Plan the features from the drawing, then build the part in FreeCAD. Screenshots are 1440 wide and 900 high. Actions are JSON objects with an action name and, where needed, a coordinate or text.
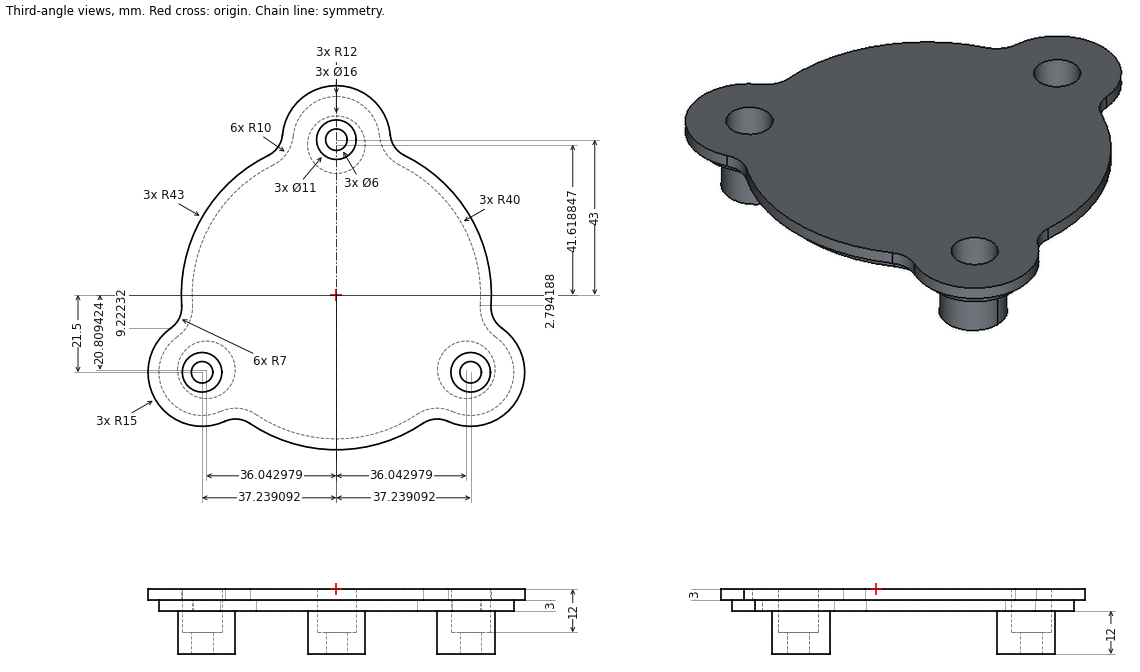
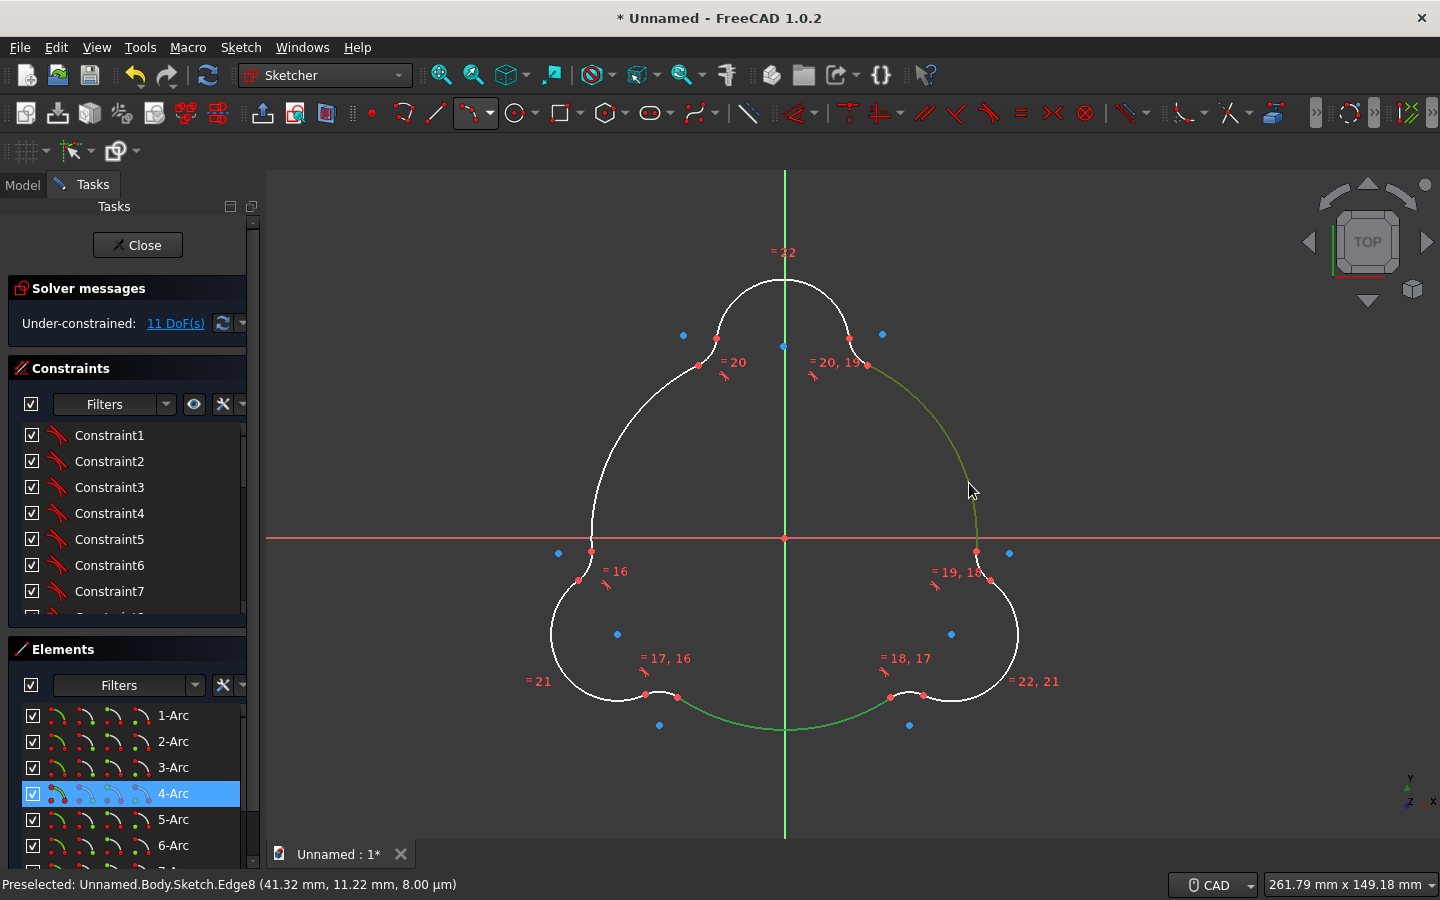
{"action": "left_click", "coordinate": [644, 406]}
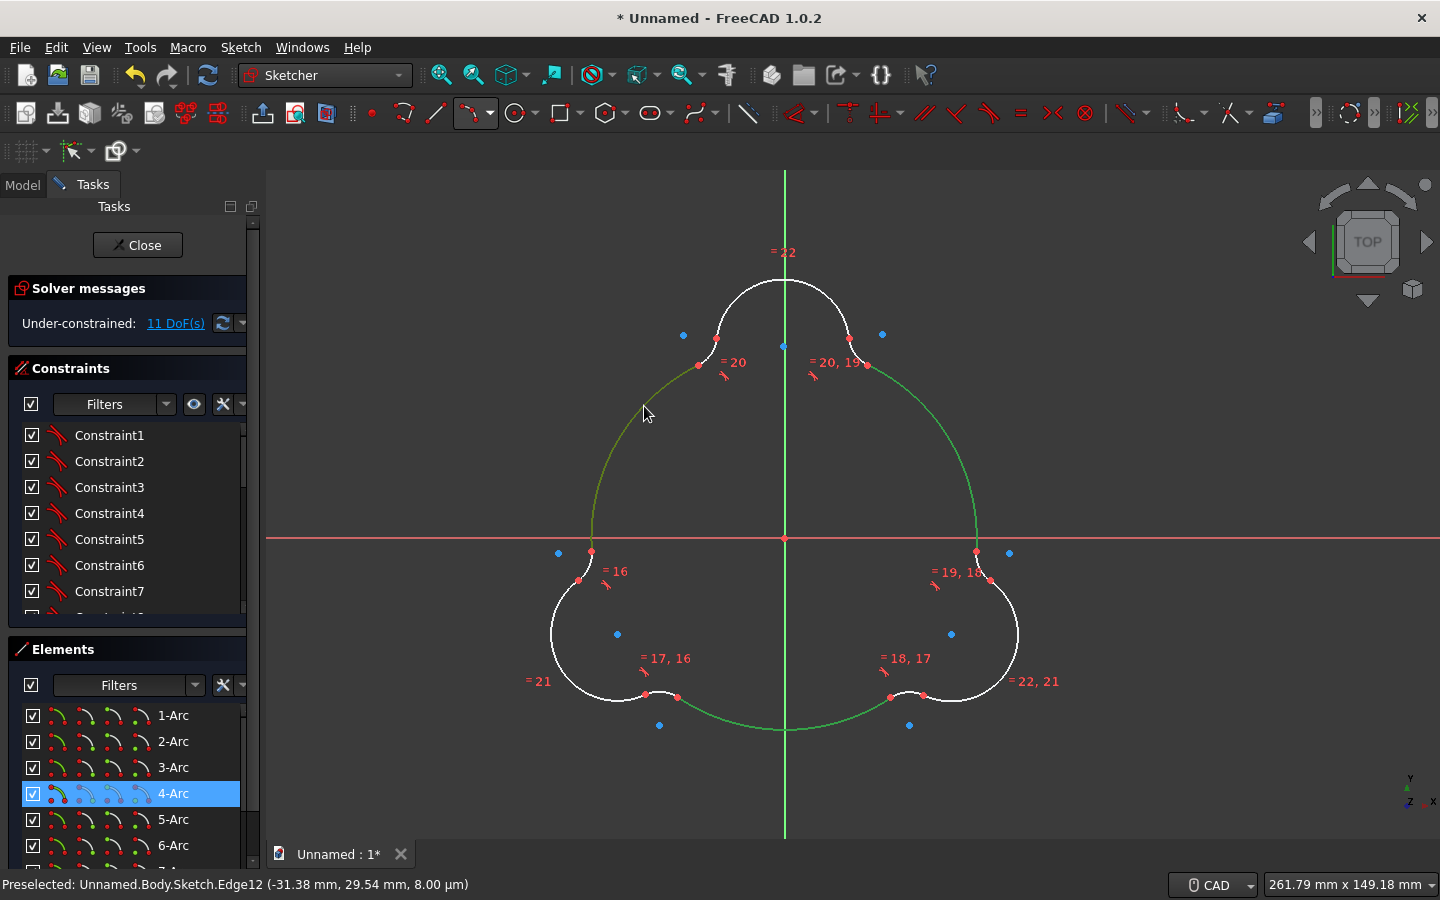
{"action": "left_click", "coordinate": [1022, 114]}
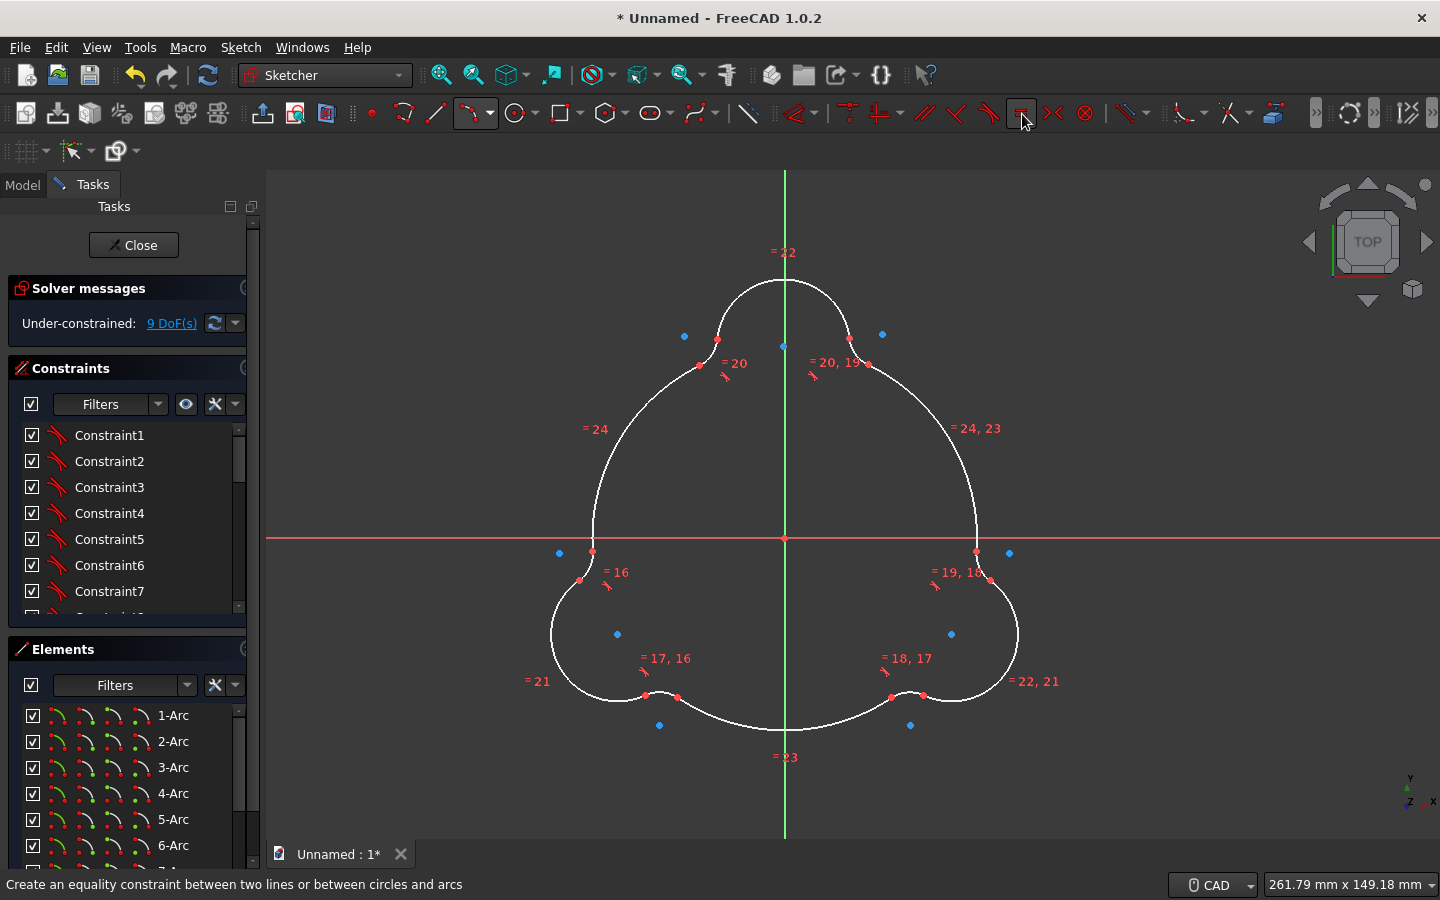
{"action": "left_click", "coordinate": [783, 346]}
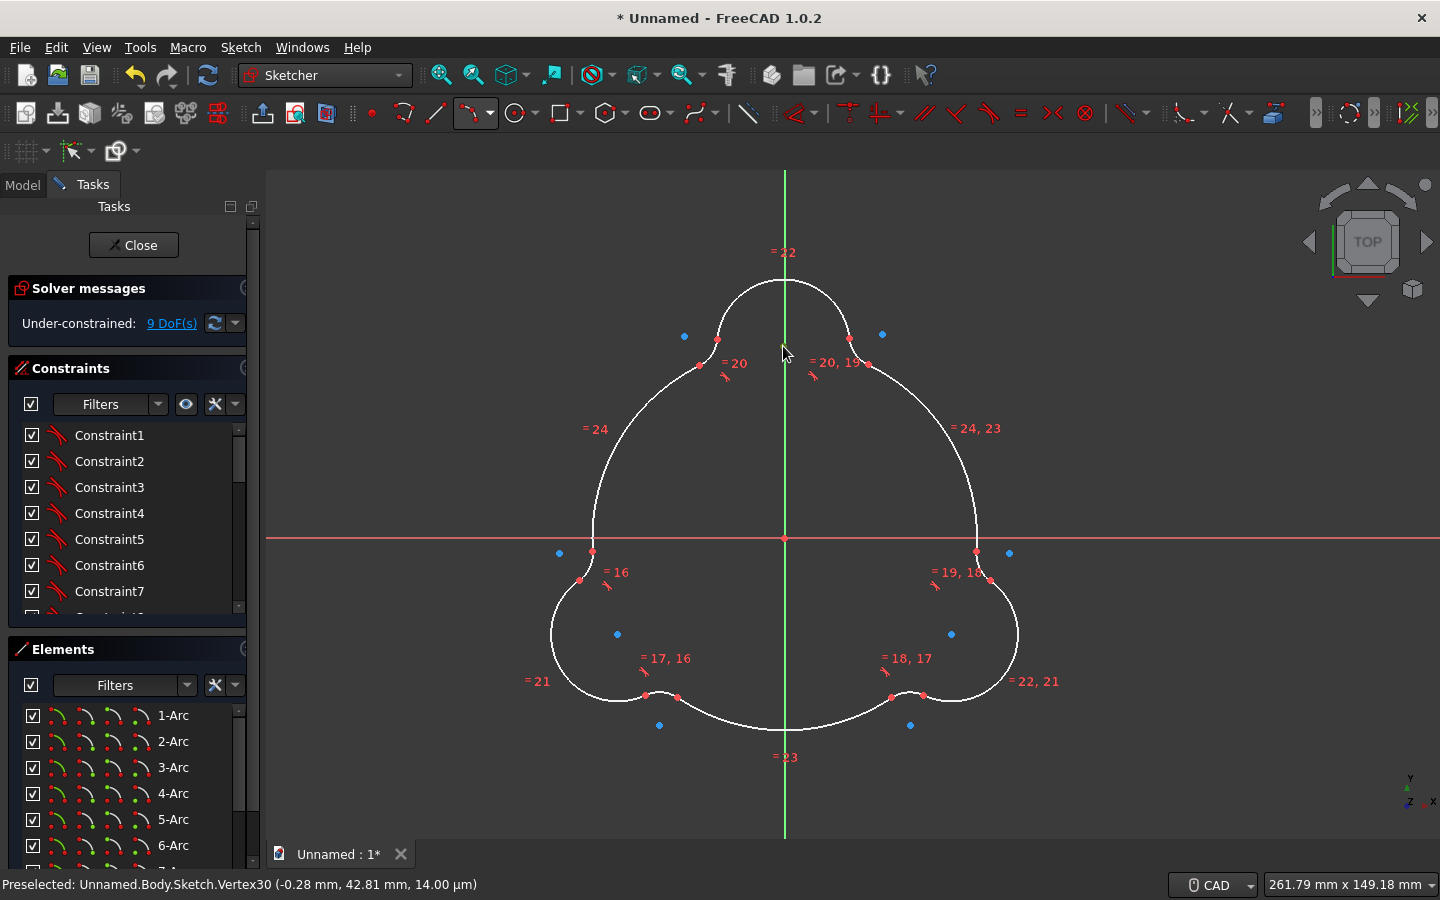
{"action": "left_click", "coordinate": [785, 767]}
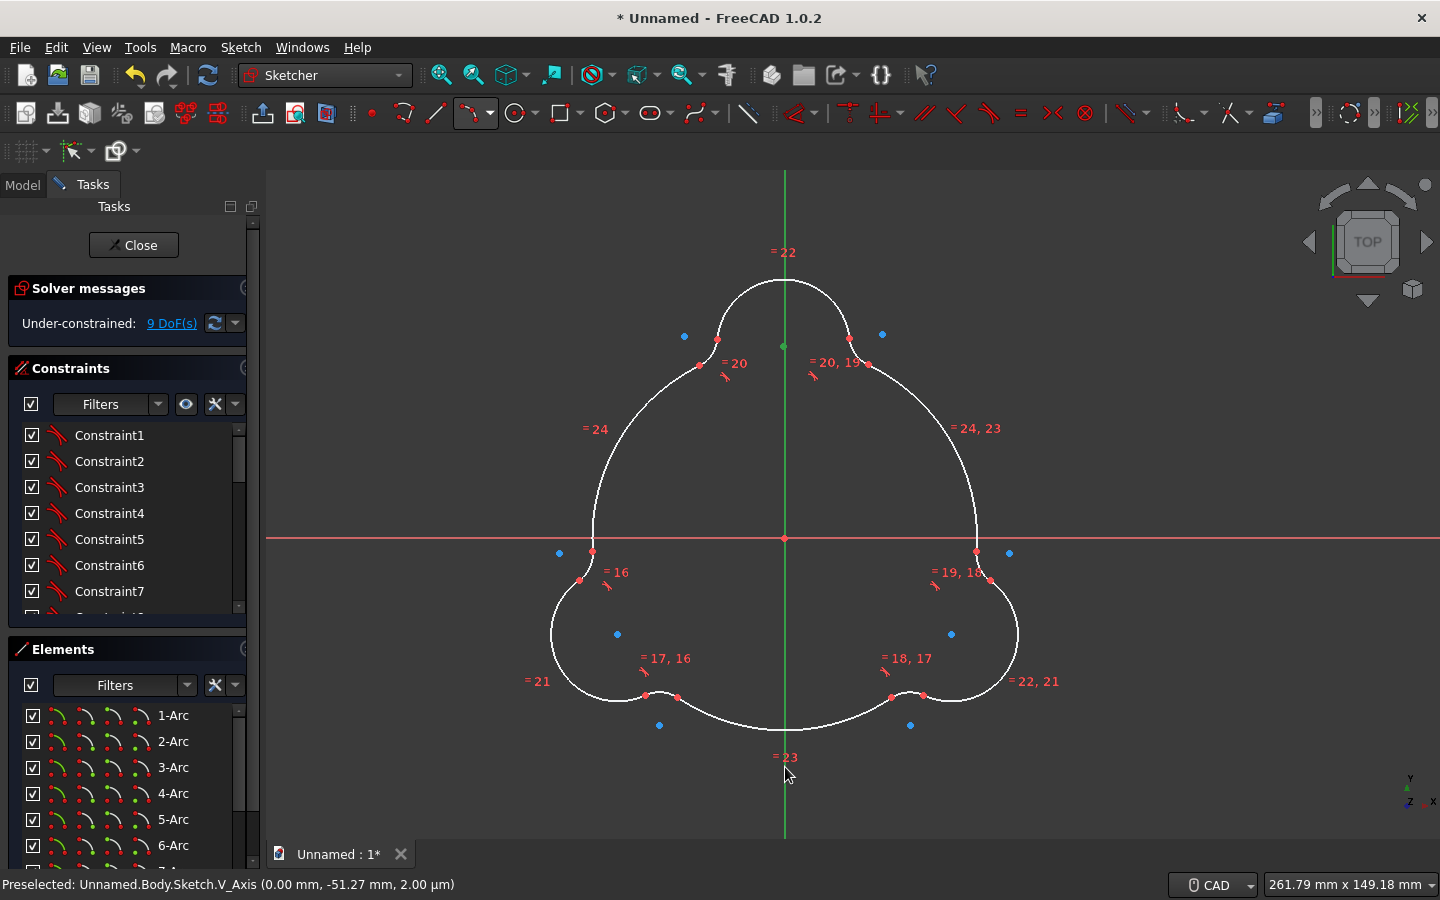
{"action": "left_click", "coordinate": [848, 114]}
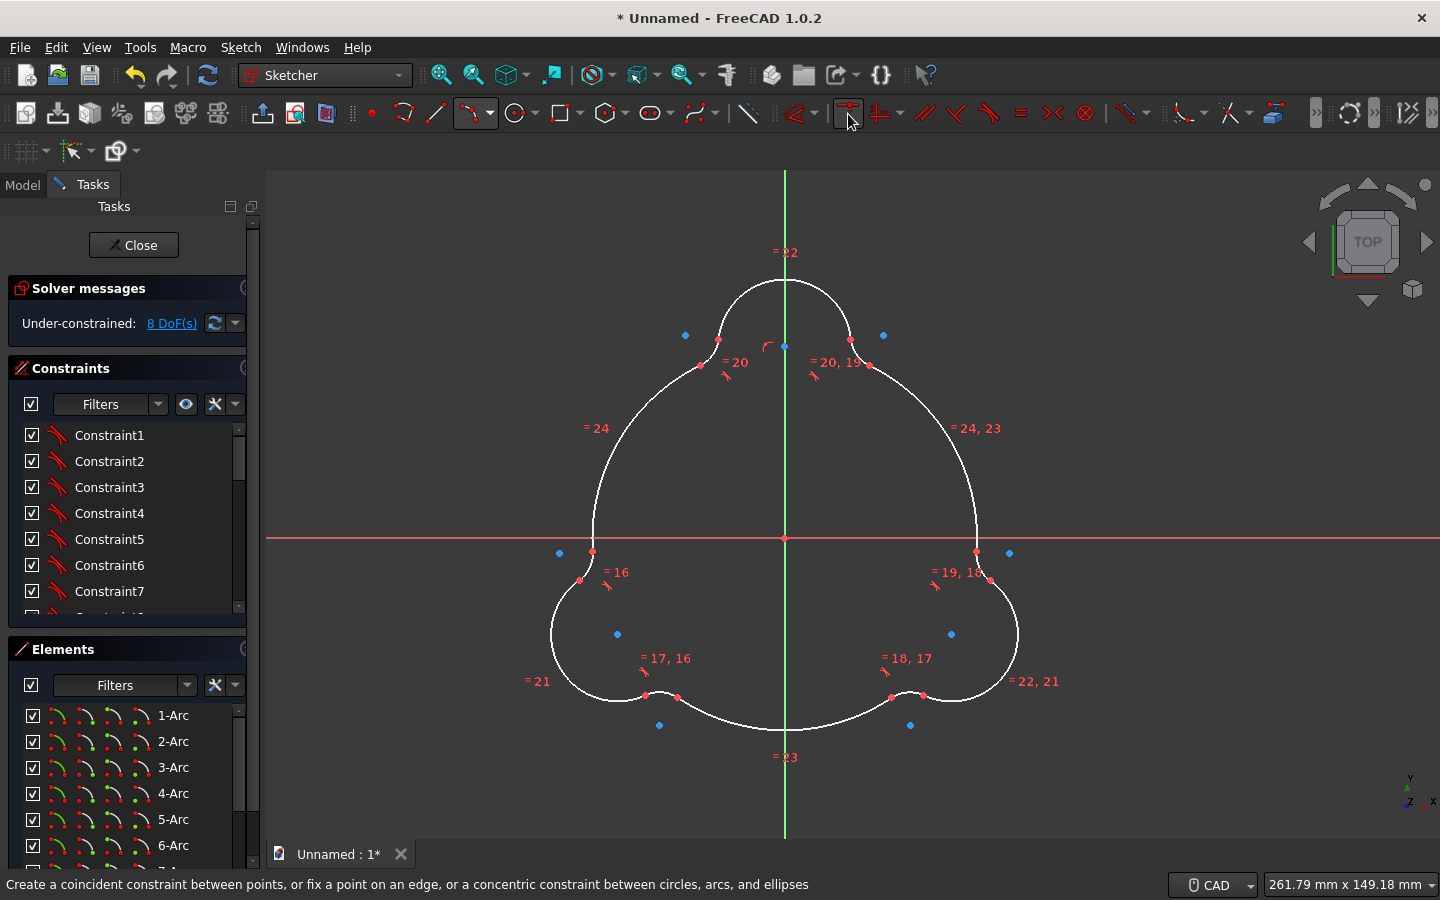
{"action": "left_click", "coordinate": [618, 635]}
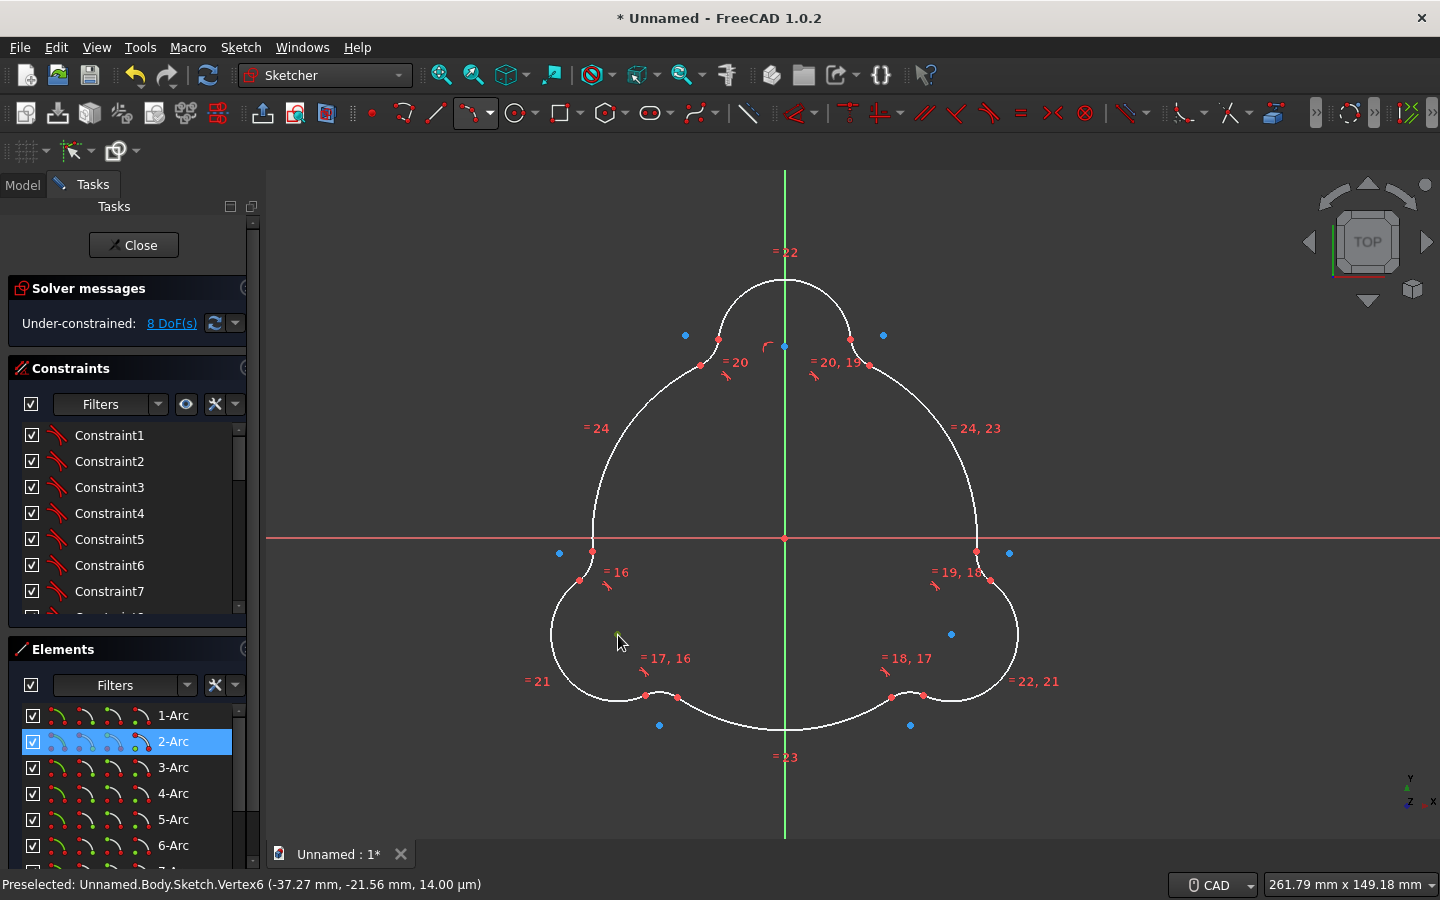
{"action": "left_click", "coordinate": [951, 635]}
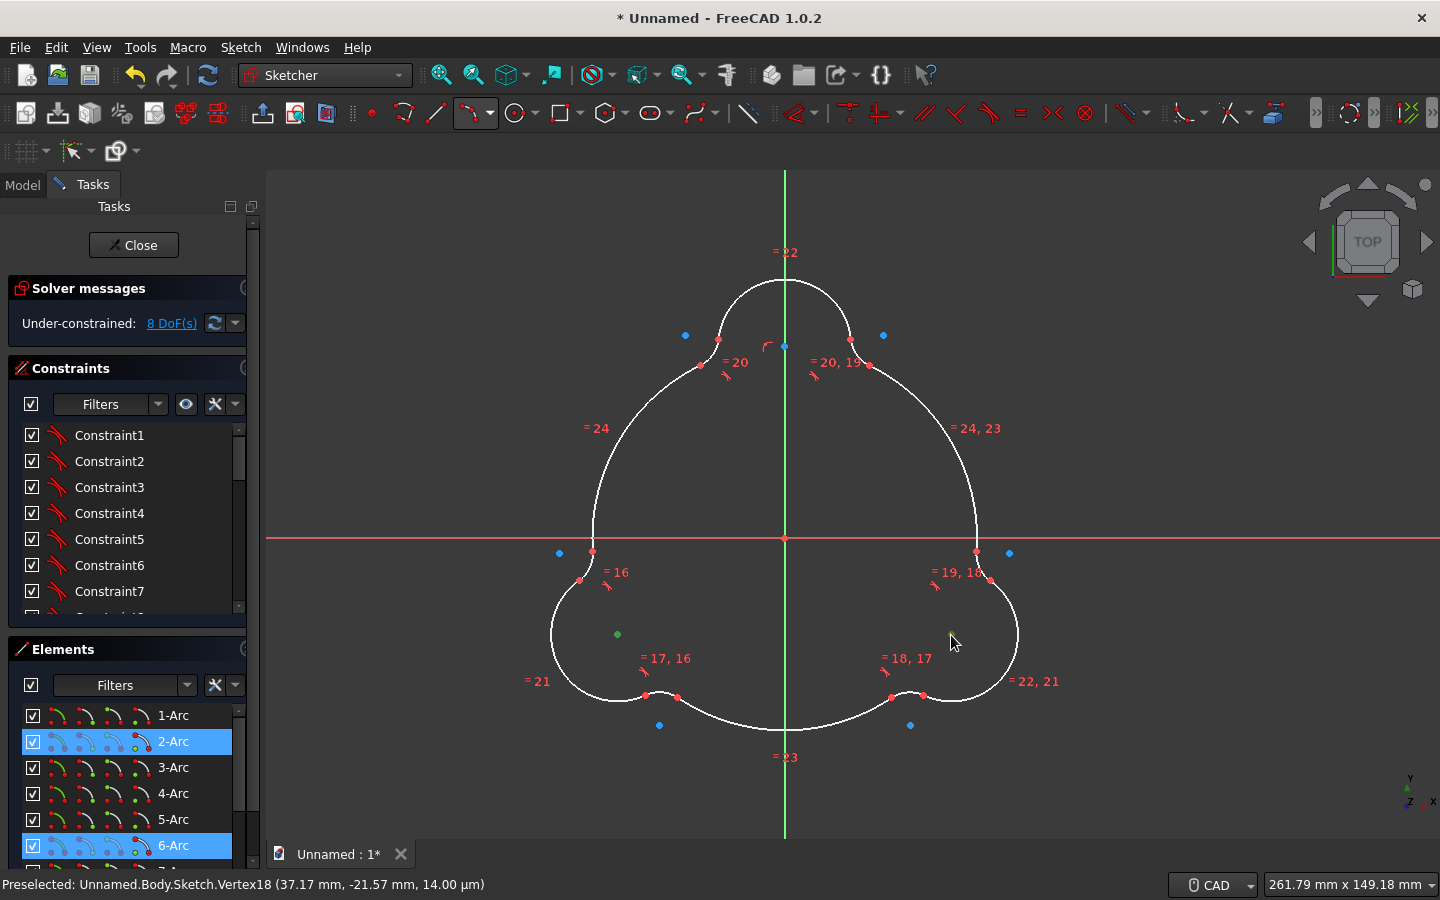
{"action": "left_click", "coordinate": [785, 767]}